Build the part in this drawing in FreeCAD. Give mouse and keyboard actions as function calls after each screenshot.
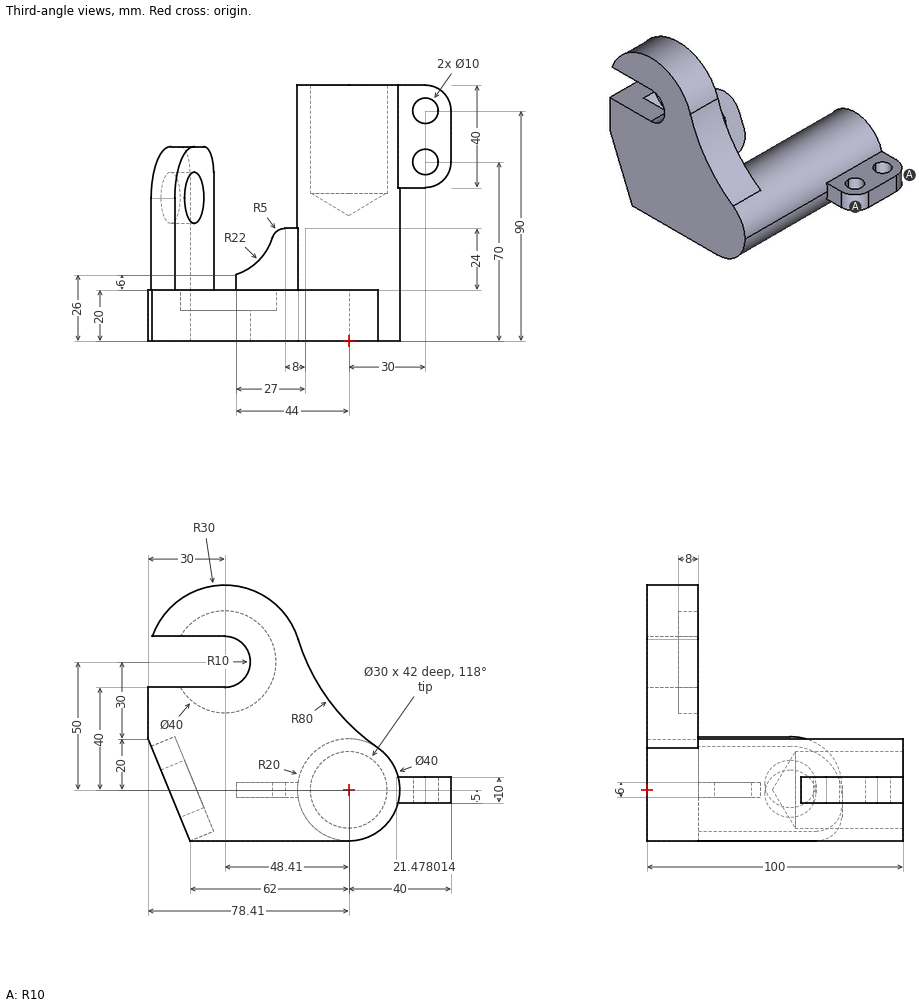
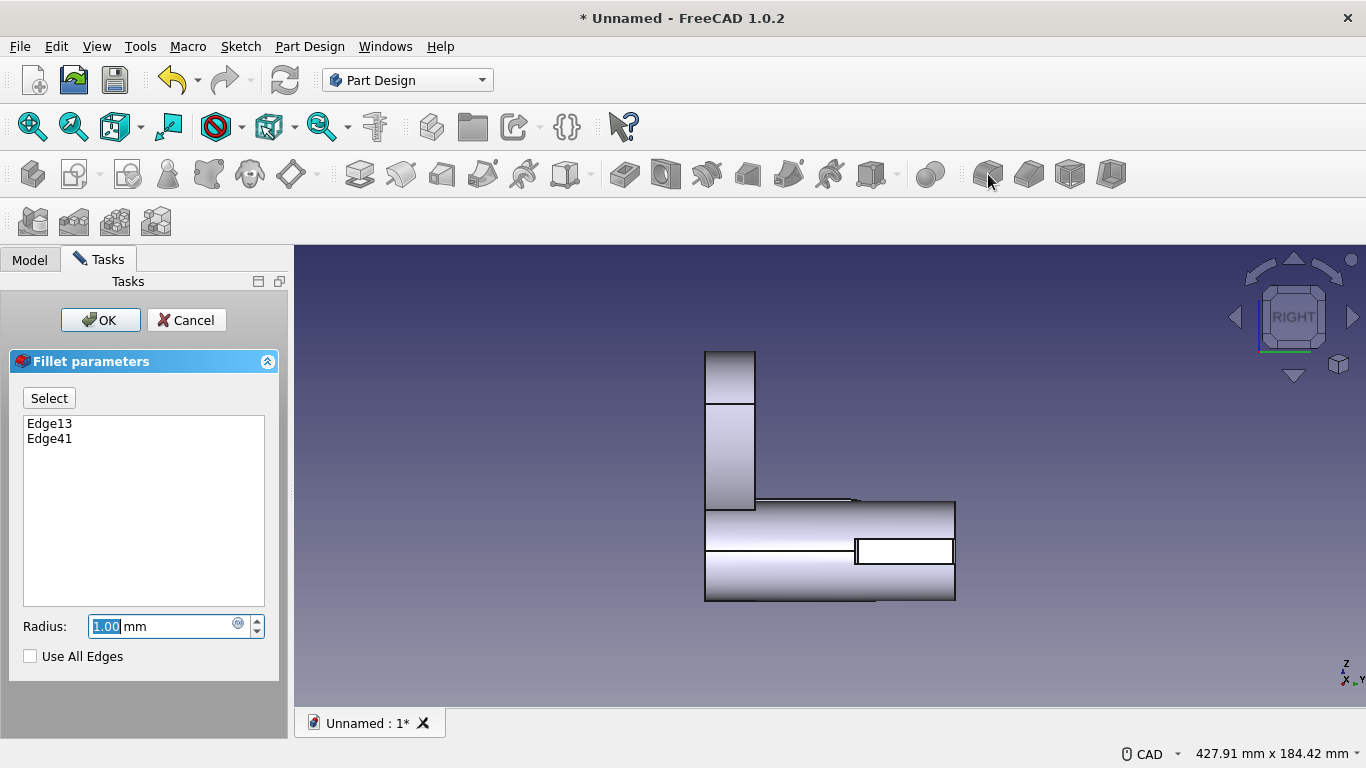
text(10)
key(Tab)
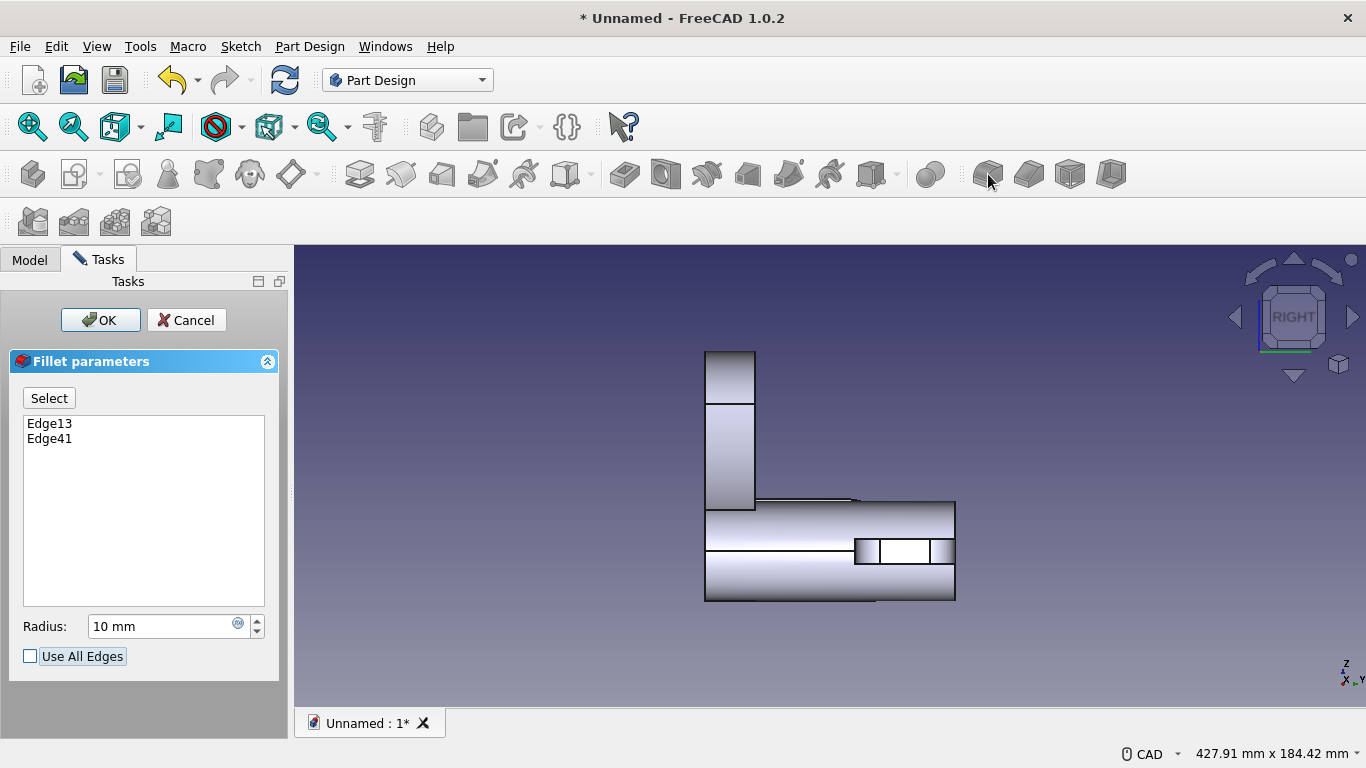
click(101, 320)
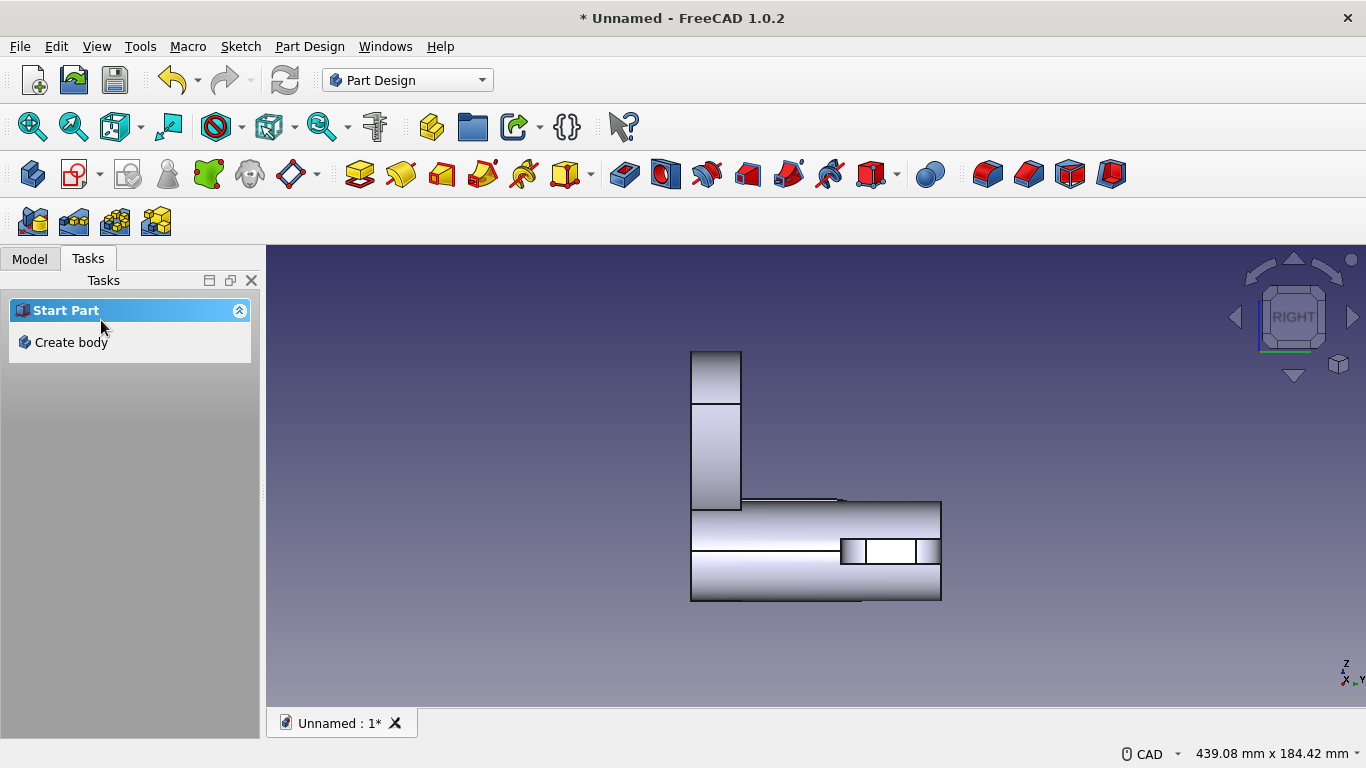
key(0)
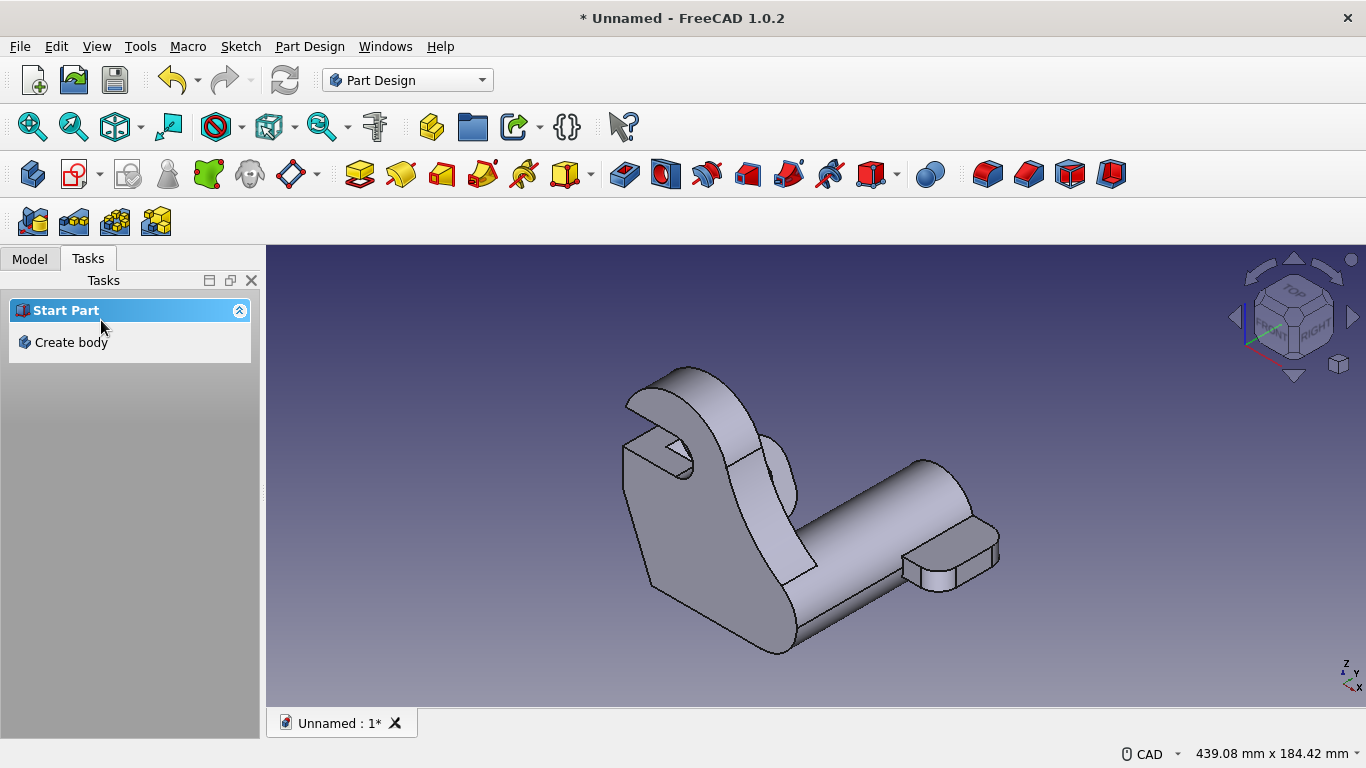
click(966, 540)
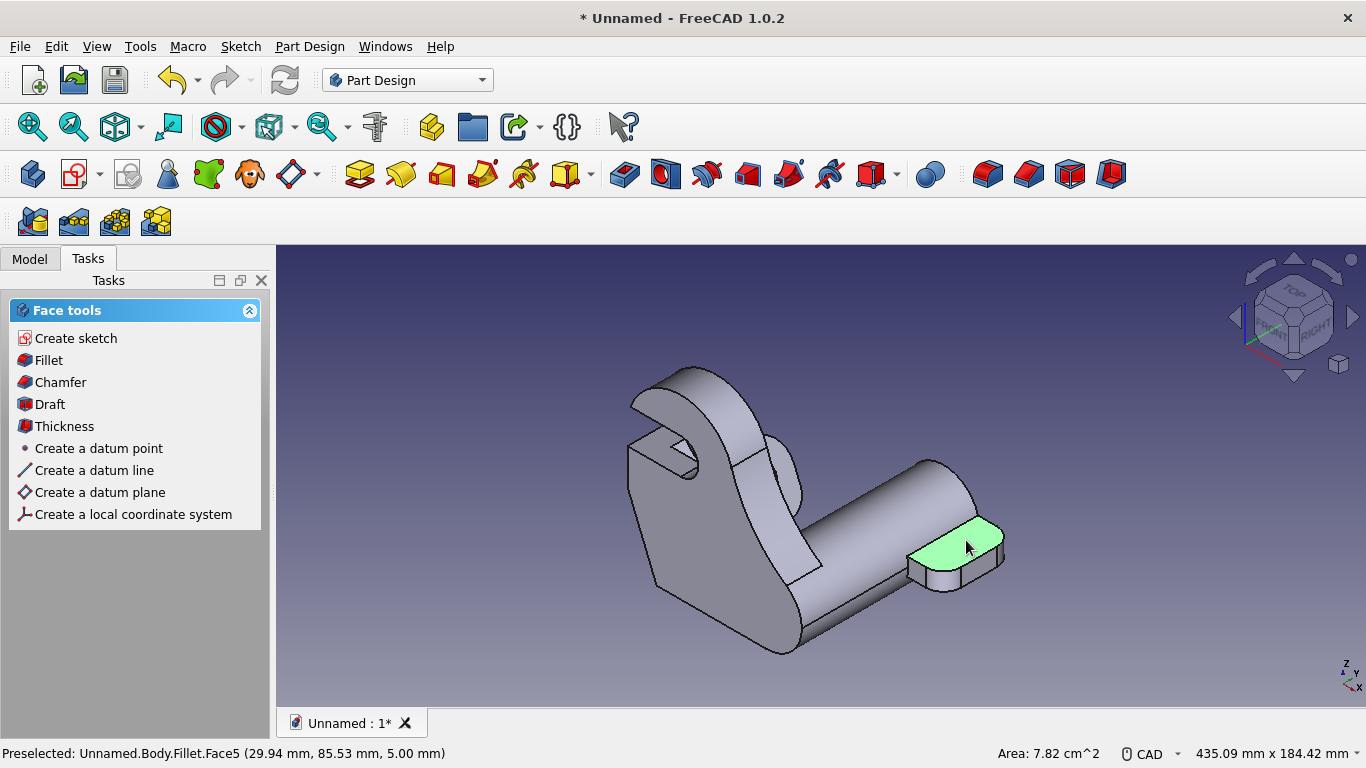
click(74, 174)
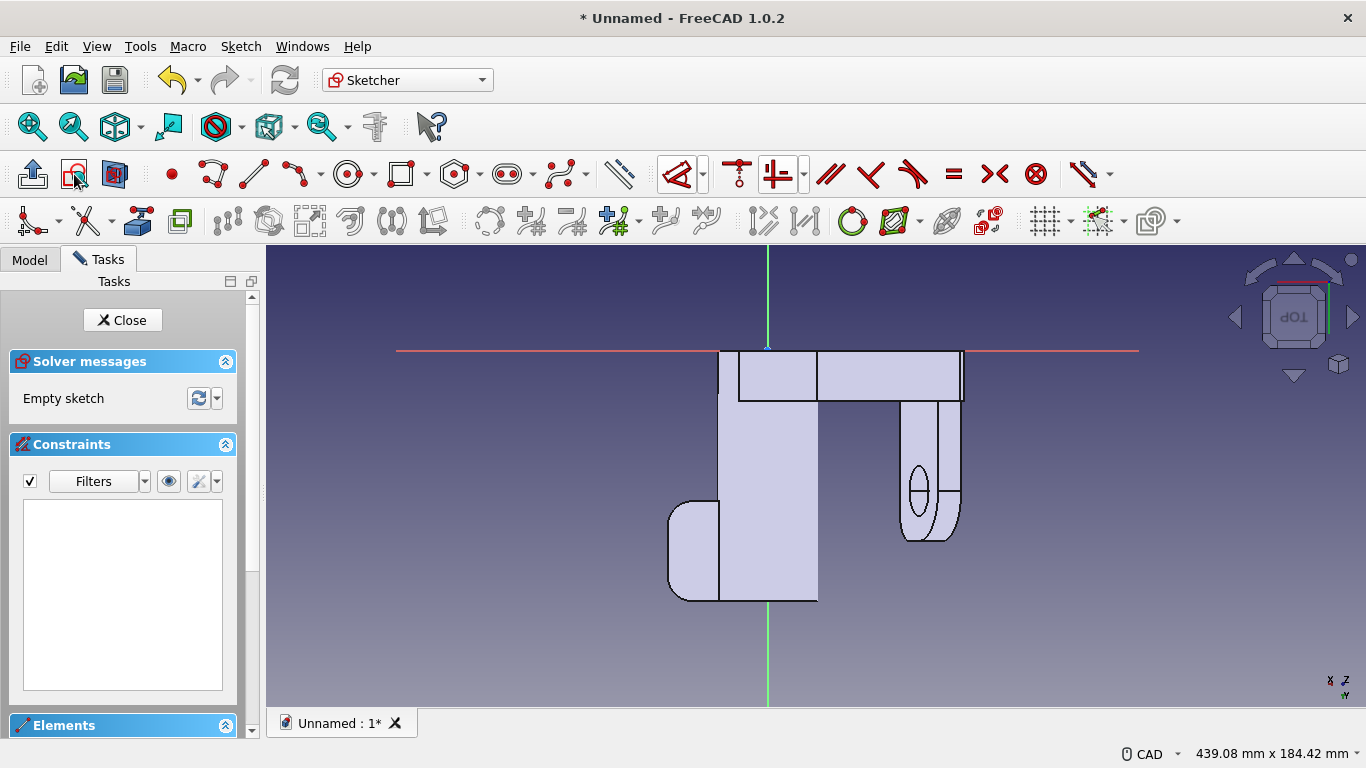
scroll(675, 576, up, 7)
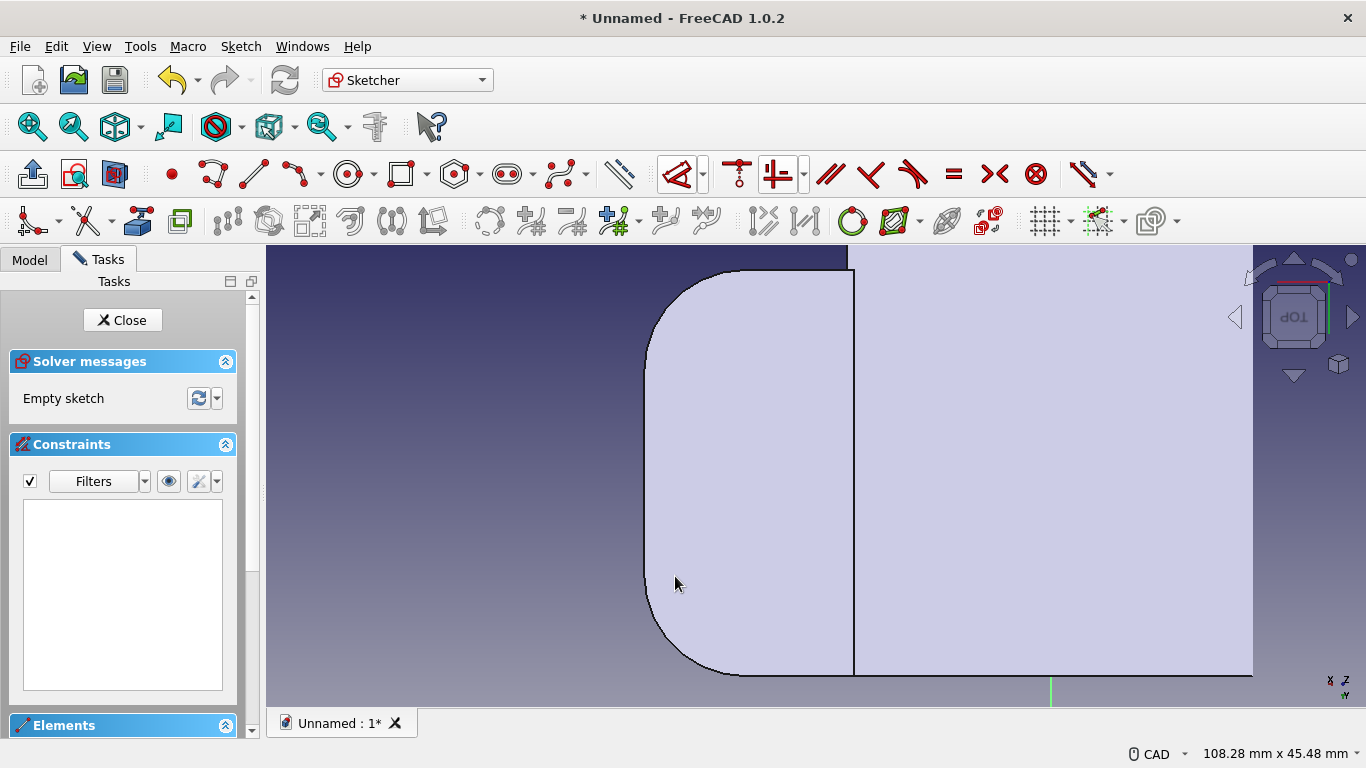
key(g)
key(c)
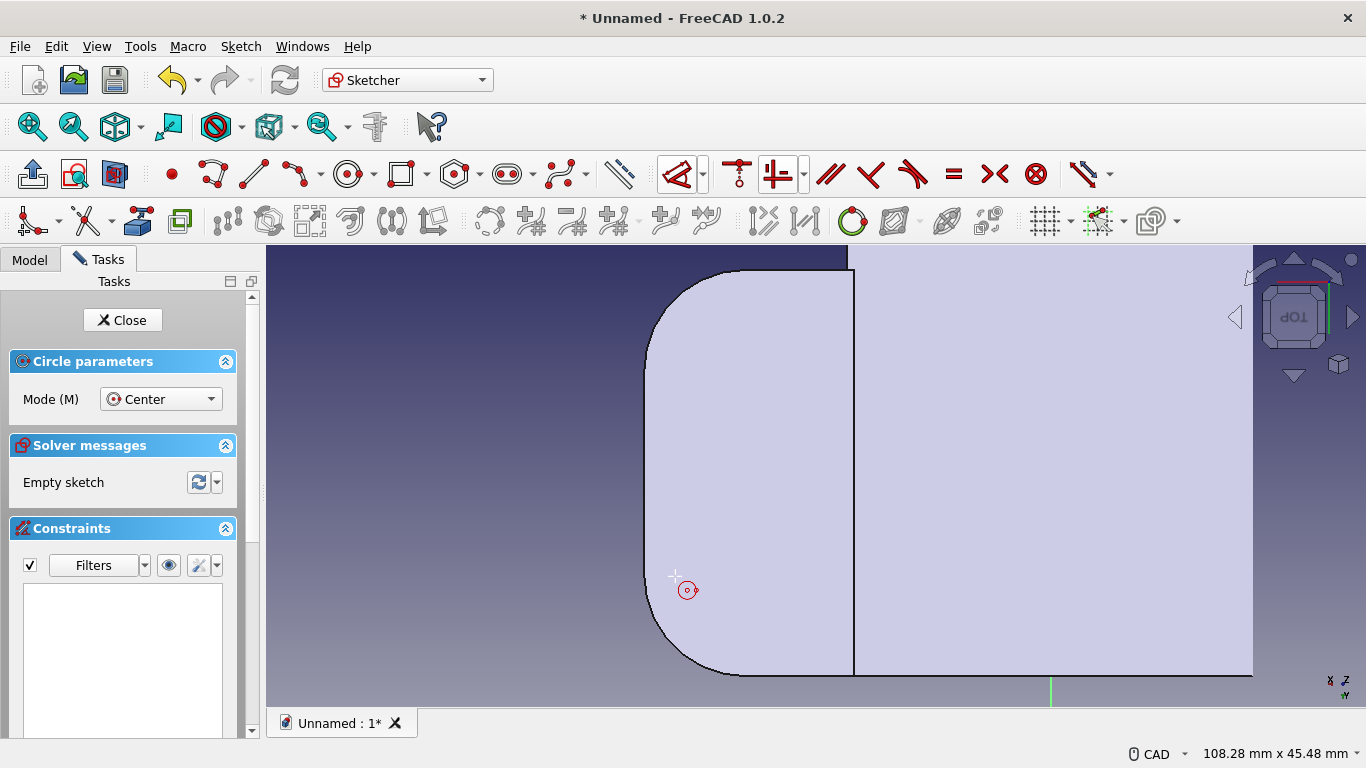
click(746, 575)
click(782, 539)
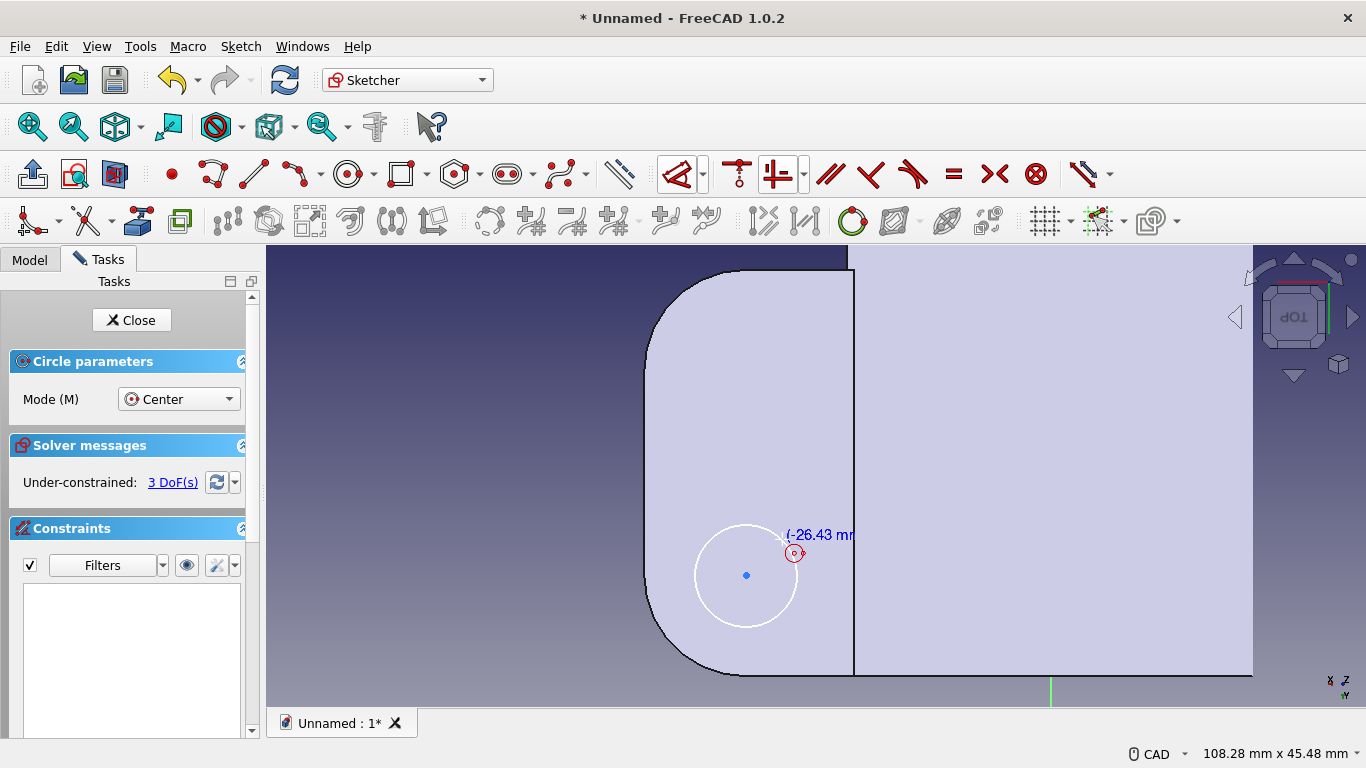
click(746, 371)
click(782, 336)
key(Escape)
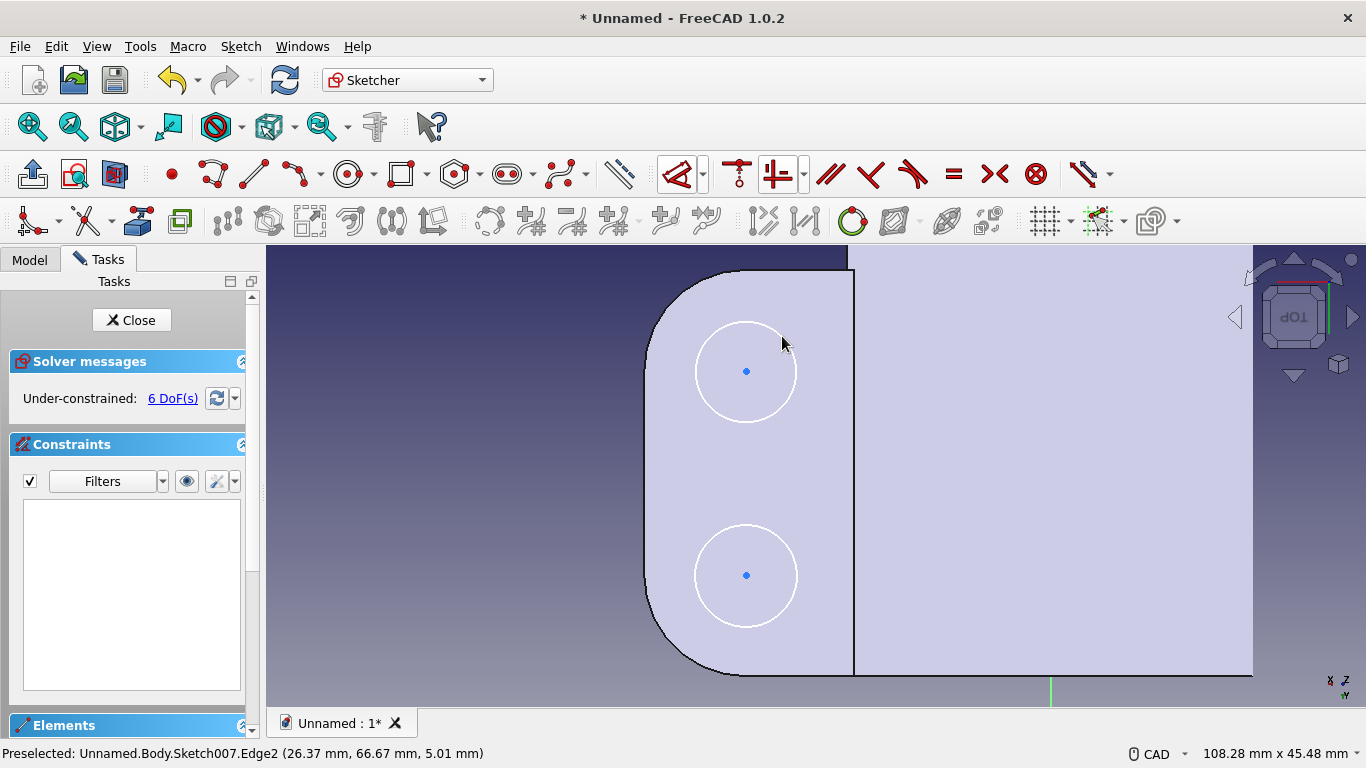
click(782, 540)